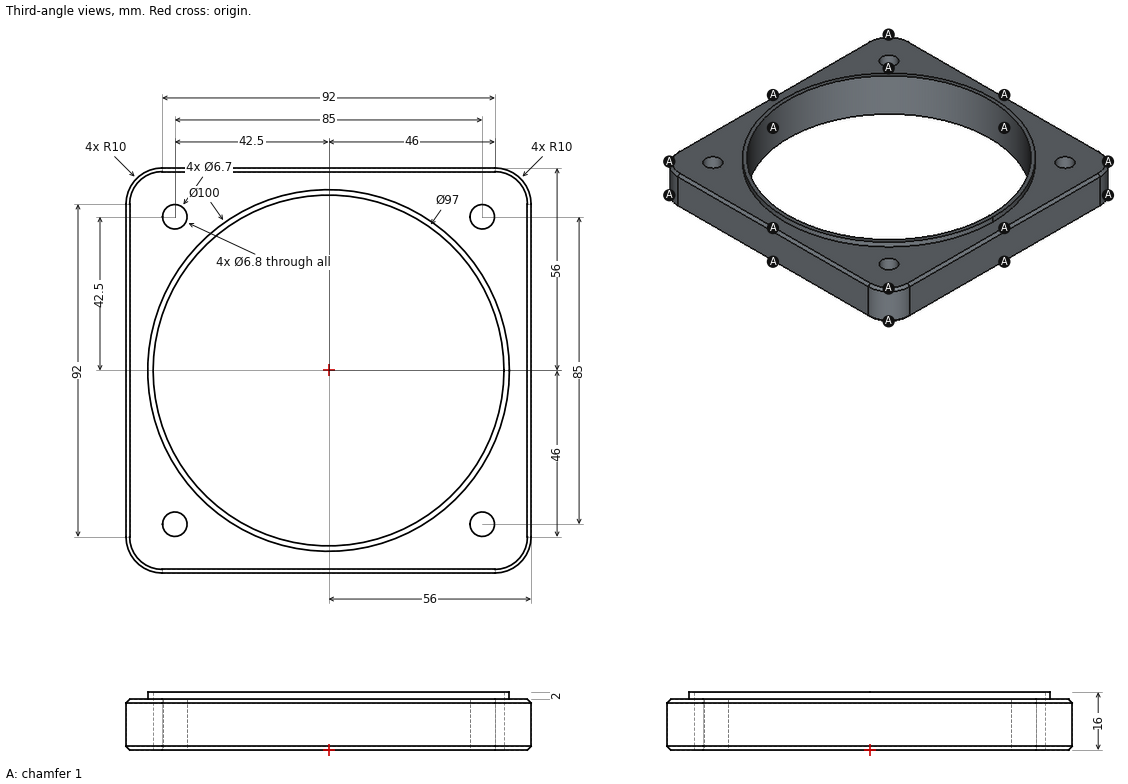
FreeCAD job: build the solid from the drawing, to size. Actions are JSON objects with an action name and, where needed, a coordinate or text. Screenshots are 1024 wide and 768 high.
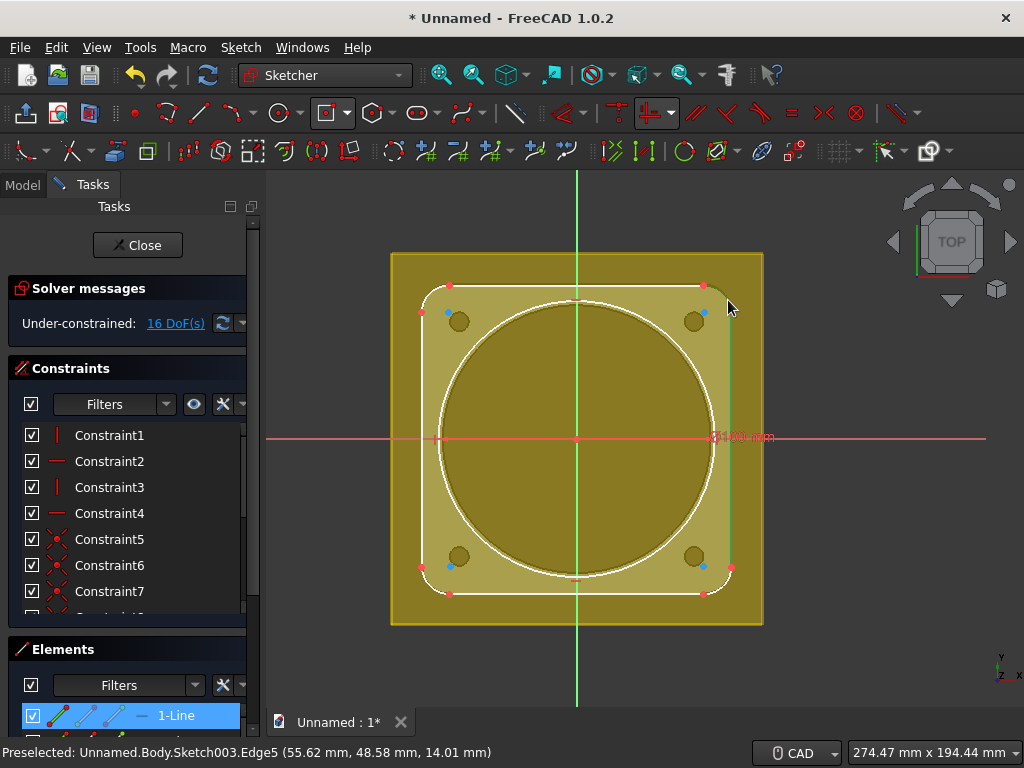
{"action": "left_click", "coordinate": [760, 114]}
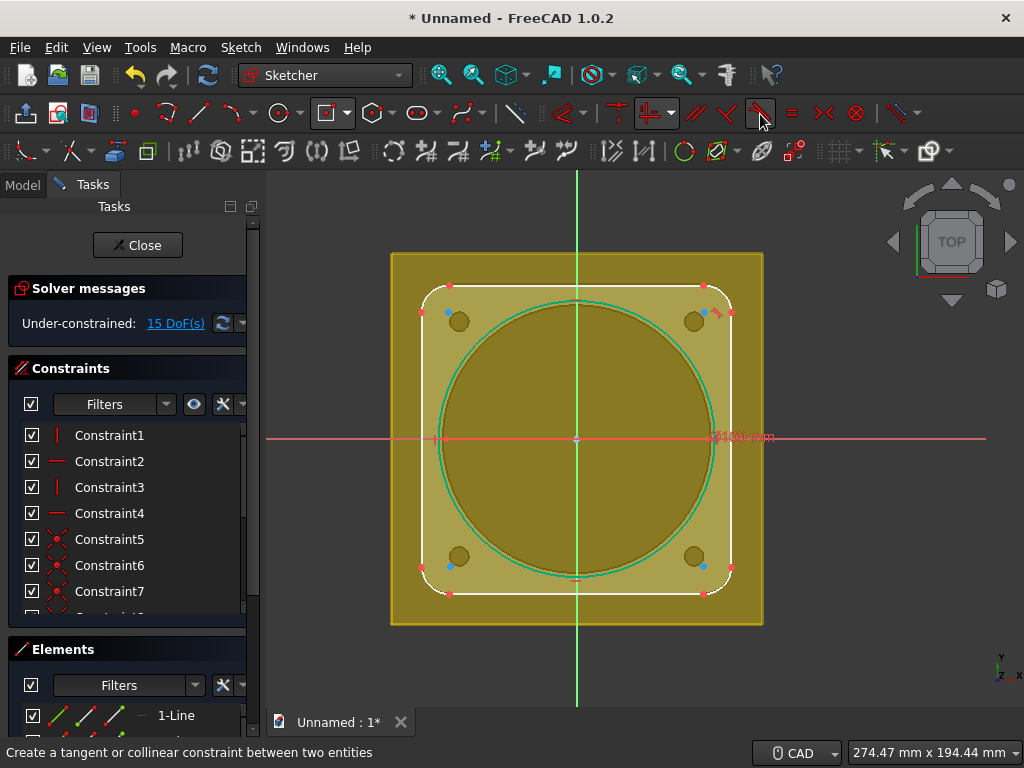
{"action": "left_click", "coordinate": [731, 491]}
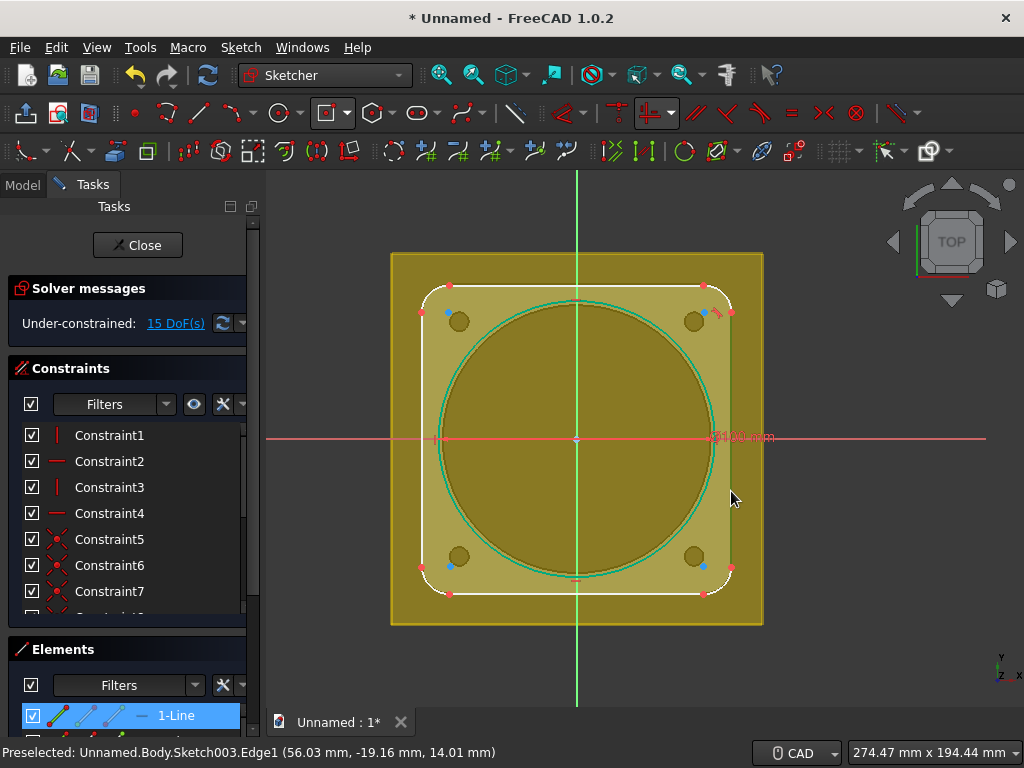
{"action": "left_click", "coordinate": [716, 591]}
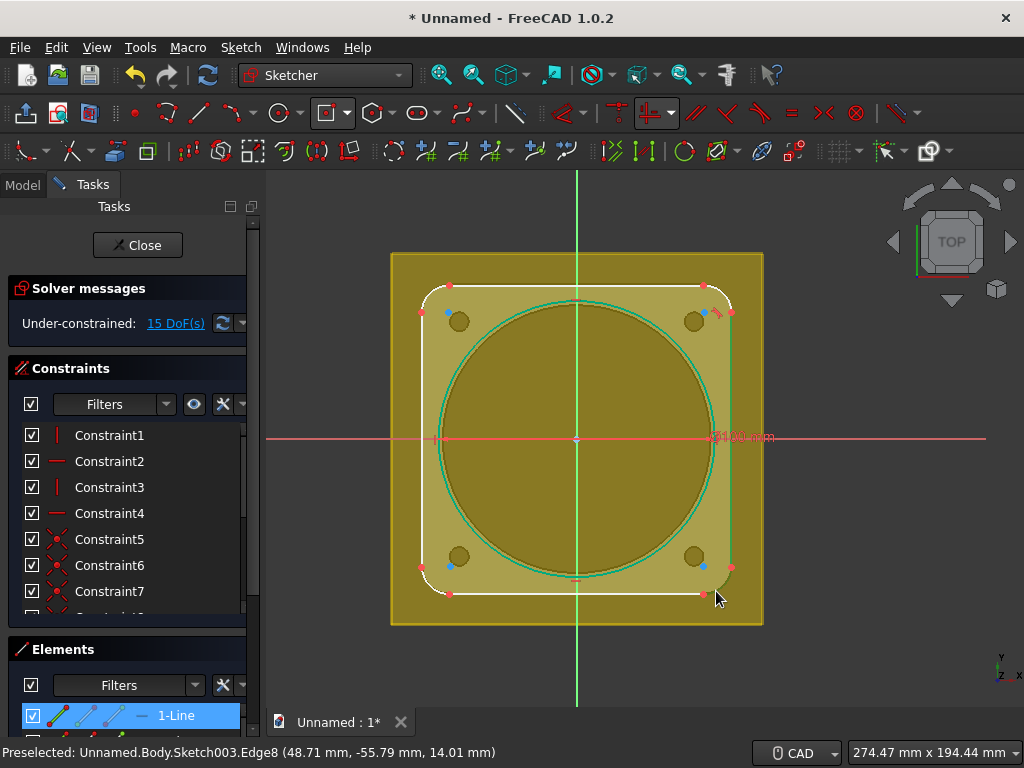
{"action": "left_click", "coordinate": [760, 114]}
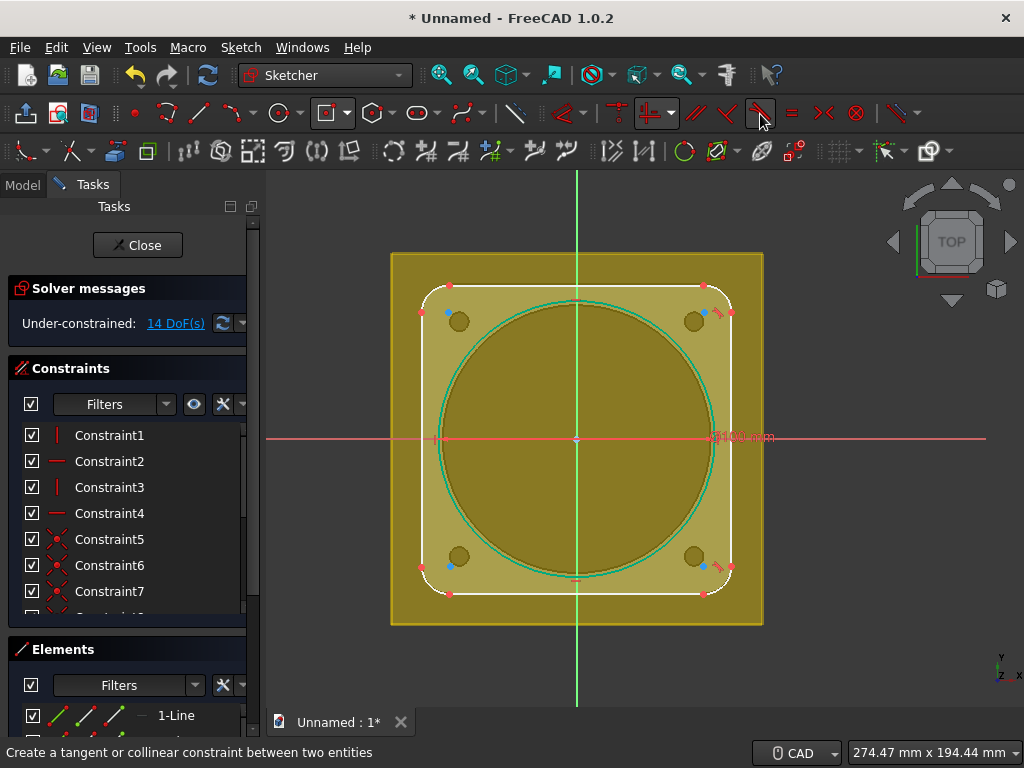
{"action": "left_click", "coordinate": [627, 286]}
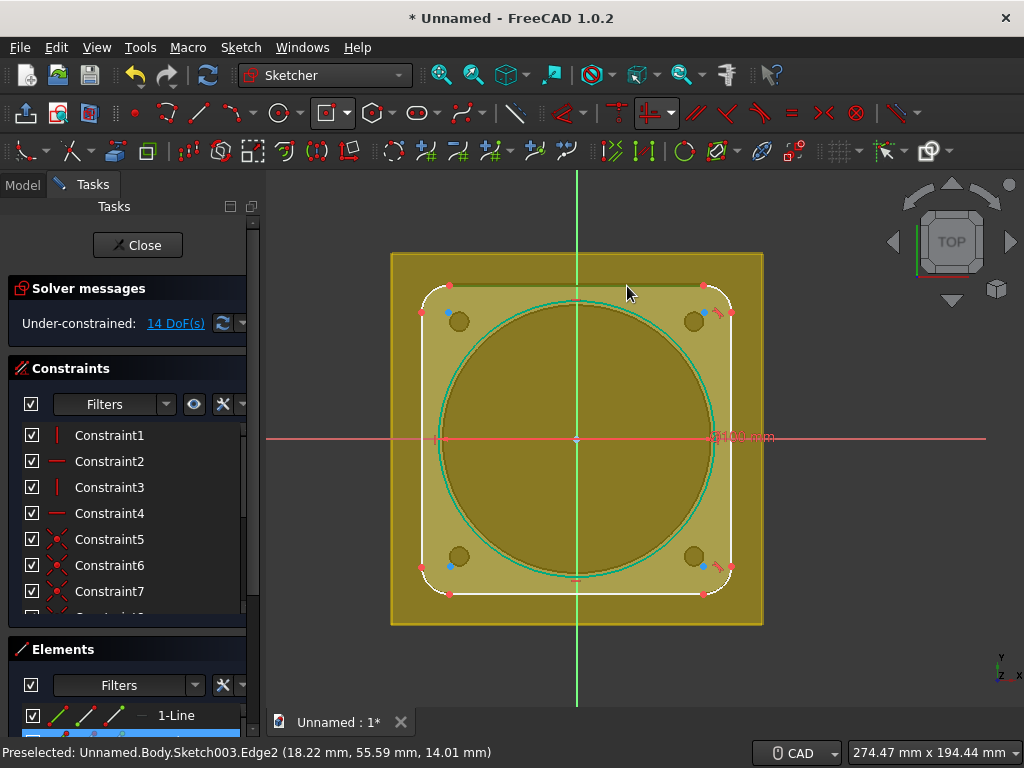
{"action": "left_click", "coordinate": [728, 300]}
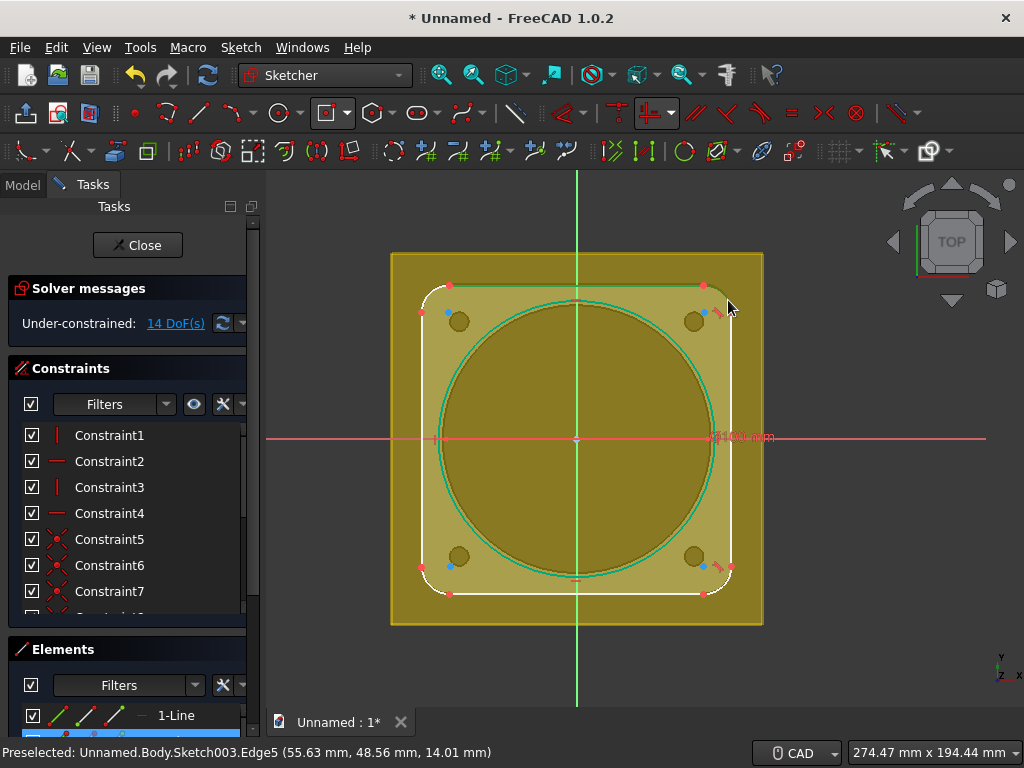
{"action": "left_click", "coordinate": [760, 114]}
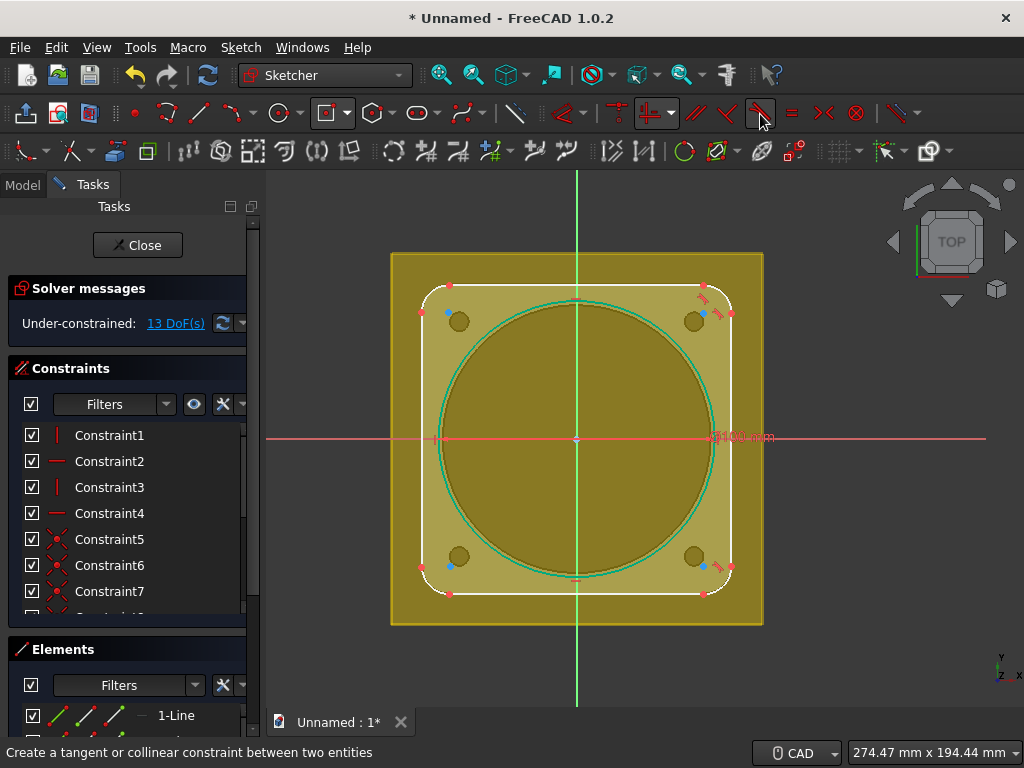
{"action": "left_click", "coordinate": [627, 285]}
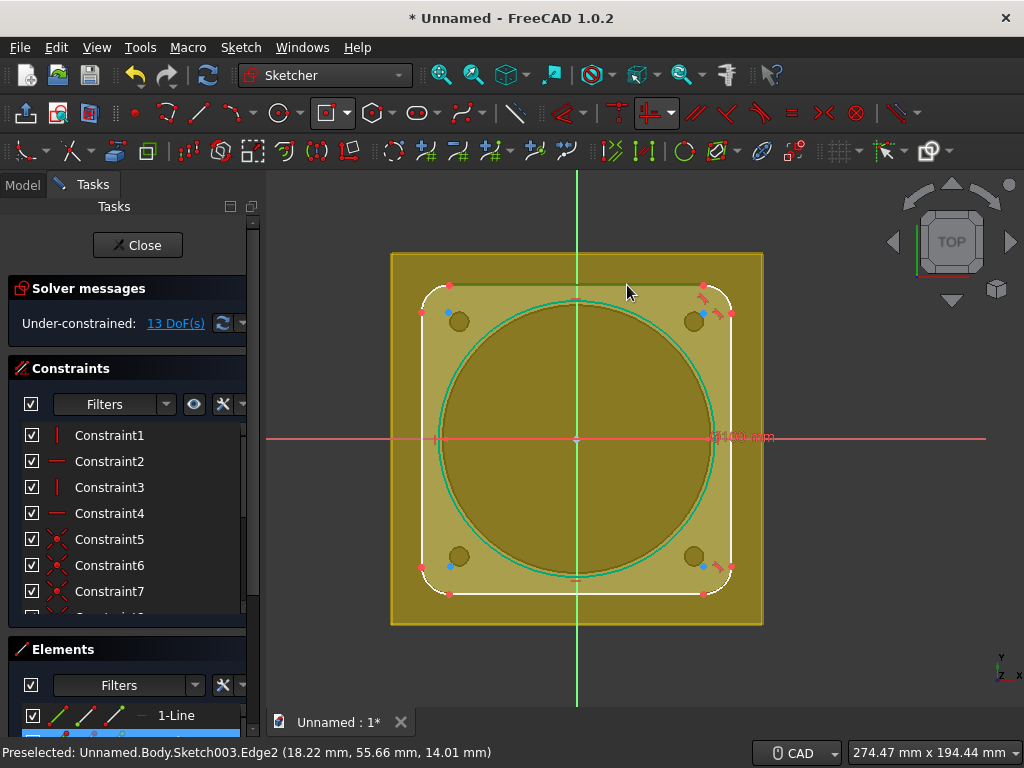
{"action": "left_click", "coordinate": [437, 288]}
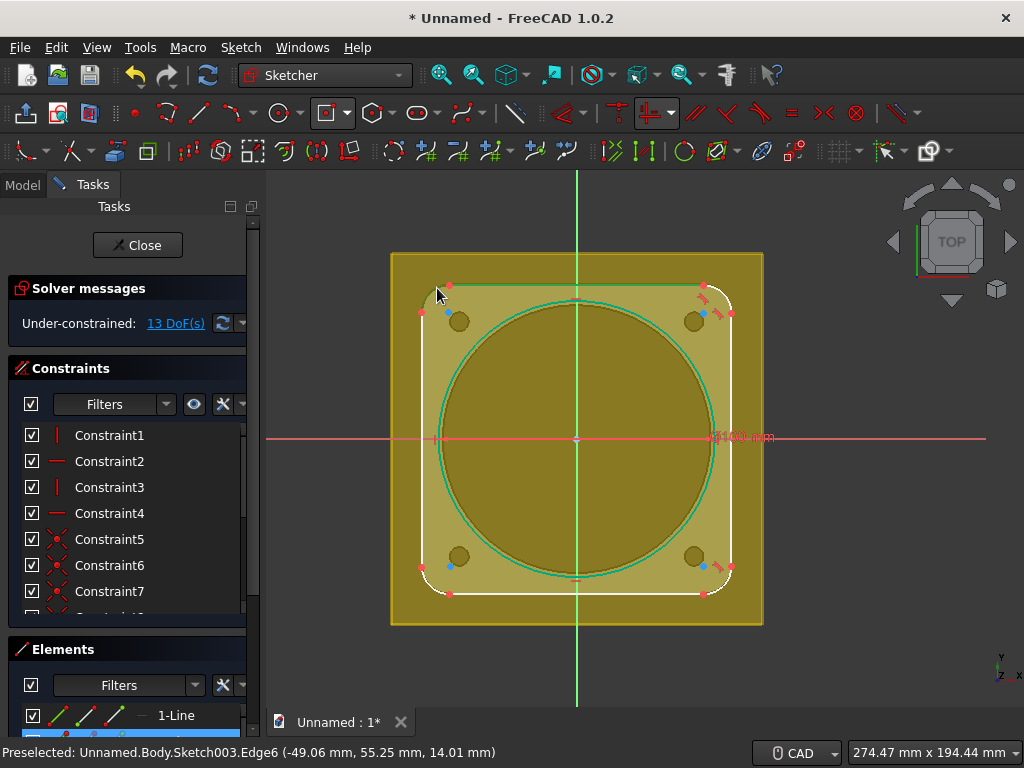
{"action": "left_click", "coordinate": [760, 114]}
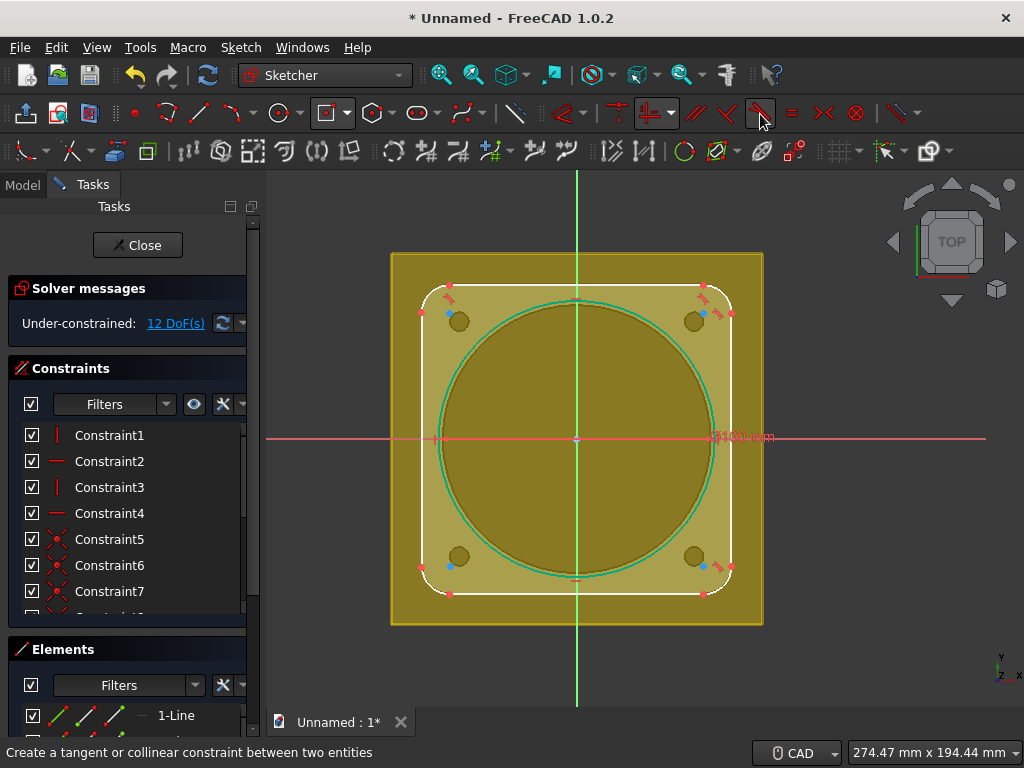
{"action": "left_click", "coordinate": [422, 389]}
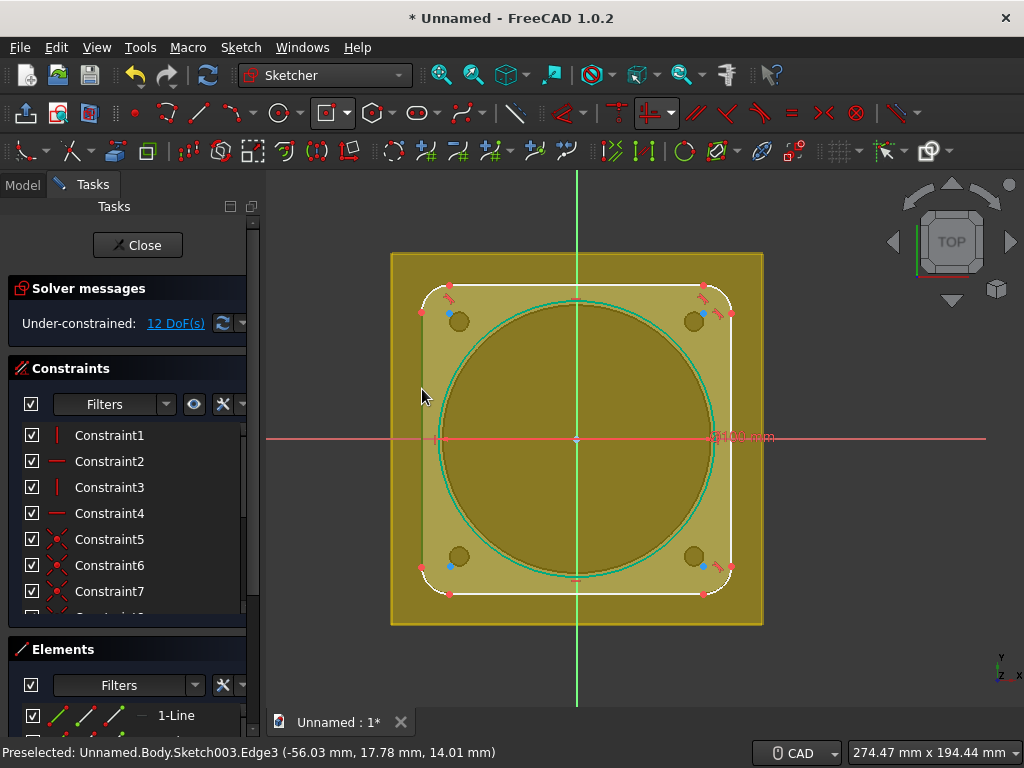
{"action": "left_click", "coordinate": [437, 288]}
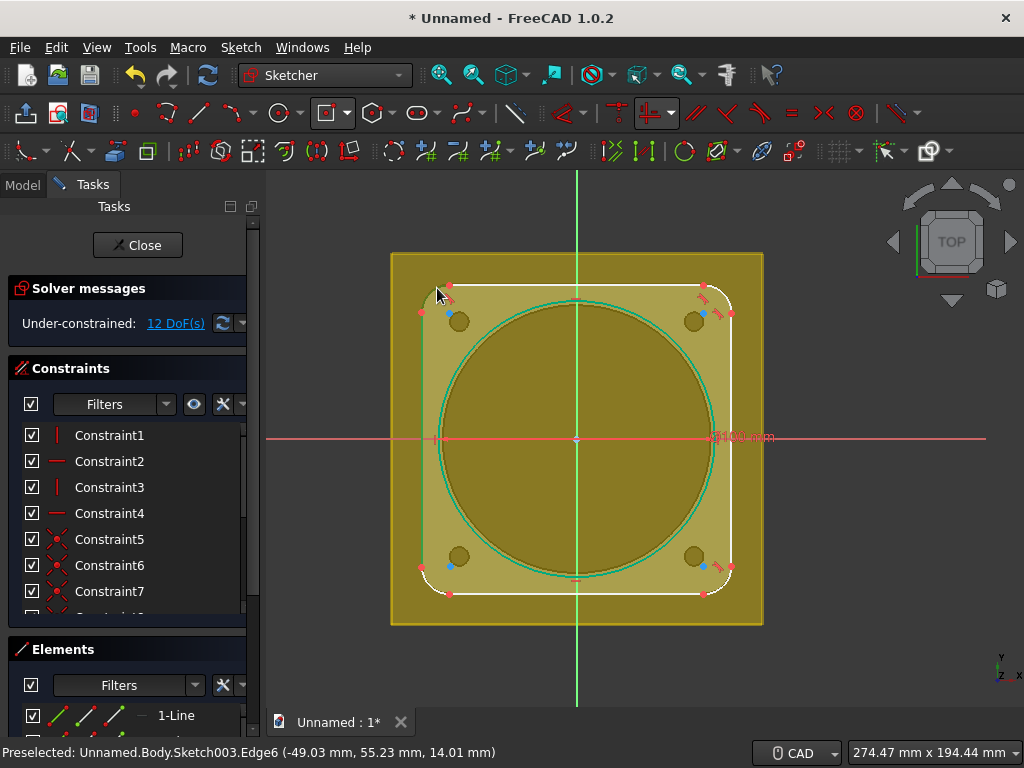
{"action": "left_click", "coordinate": [760, 114]}